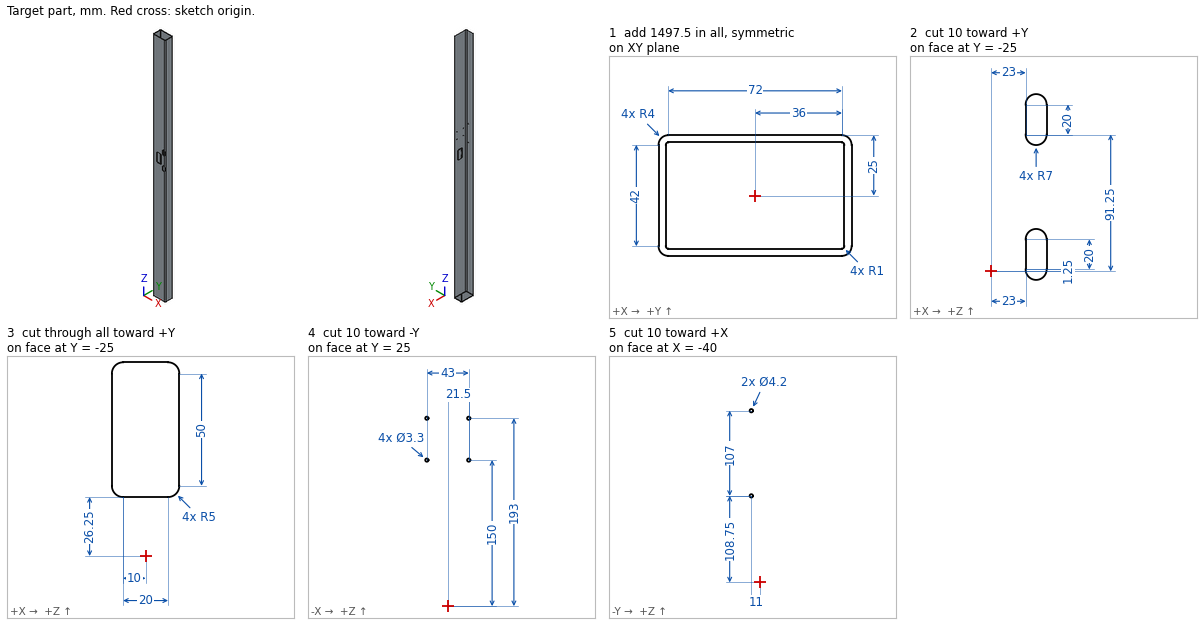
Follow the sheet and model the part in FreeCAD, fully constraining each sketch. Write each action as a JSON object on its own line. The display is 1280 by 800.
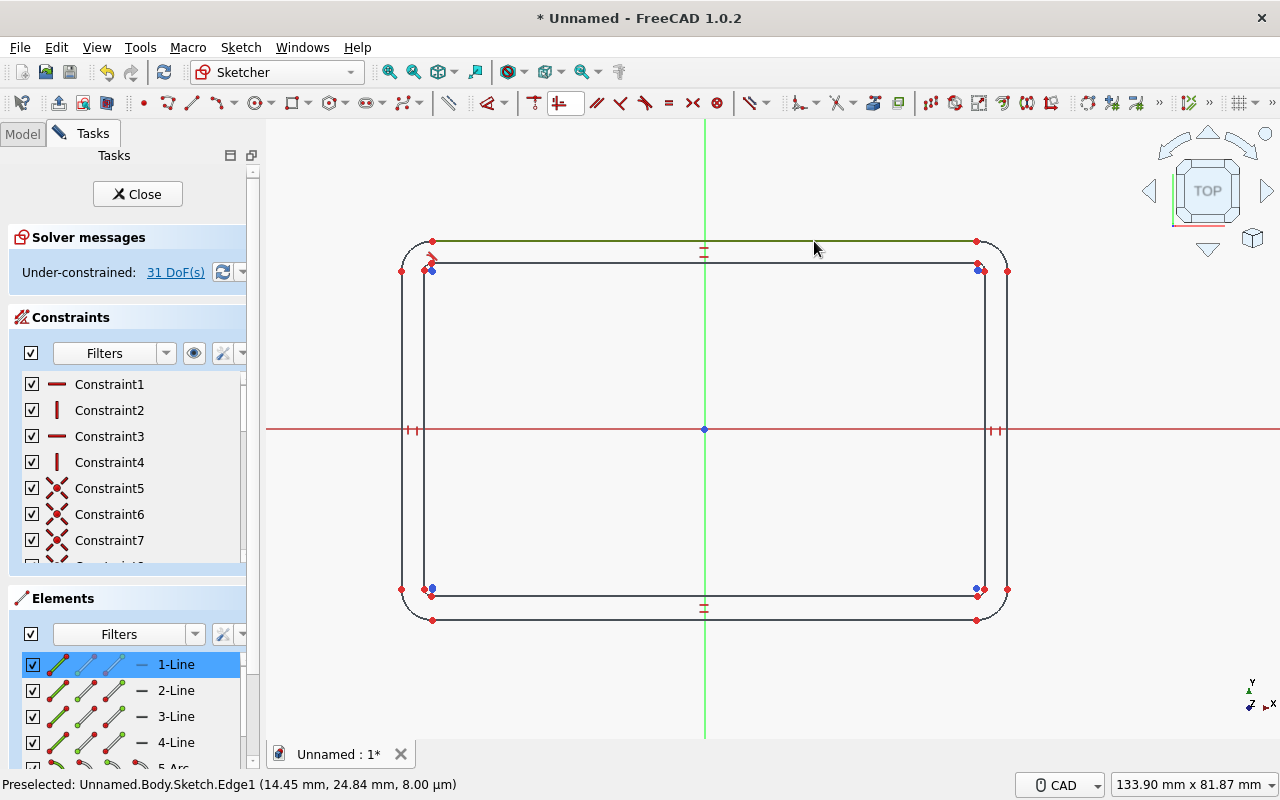
{"action": "left_click", "coordinate": [1005, 258]}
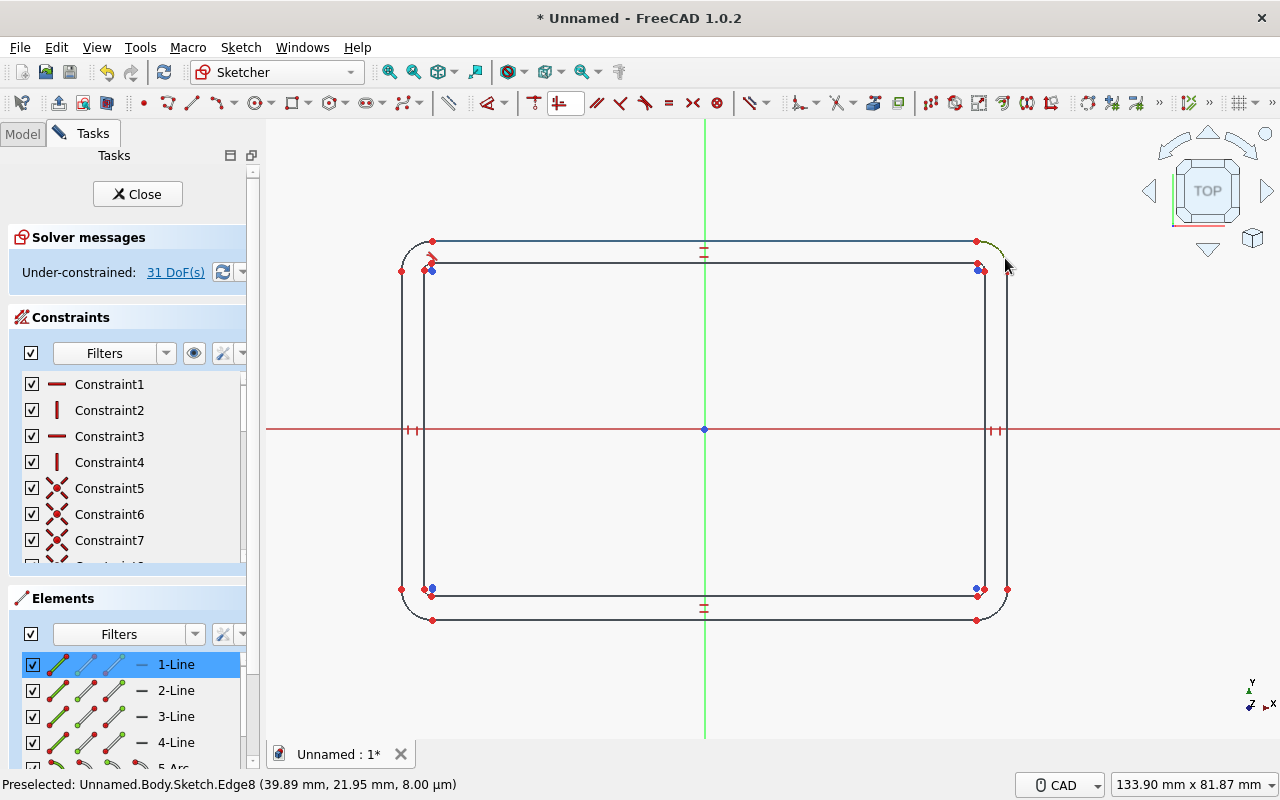
{"action": "left_click", "coordinate": [646, 104]}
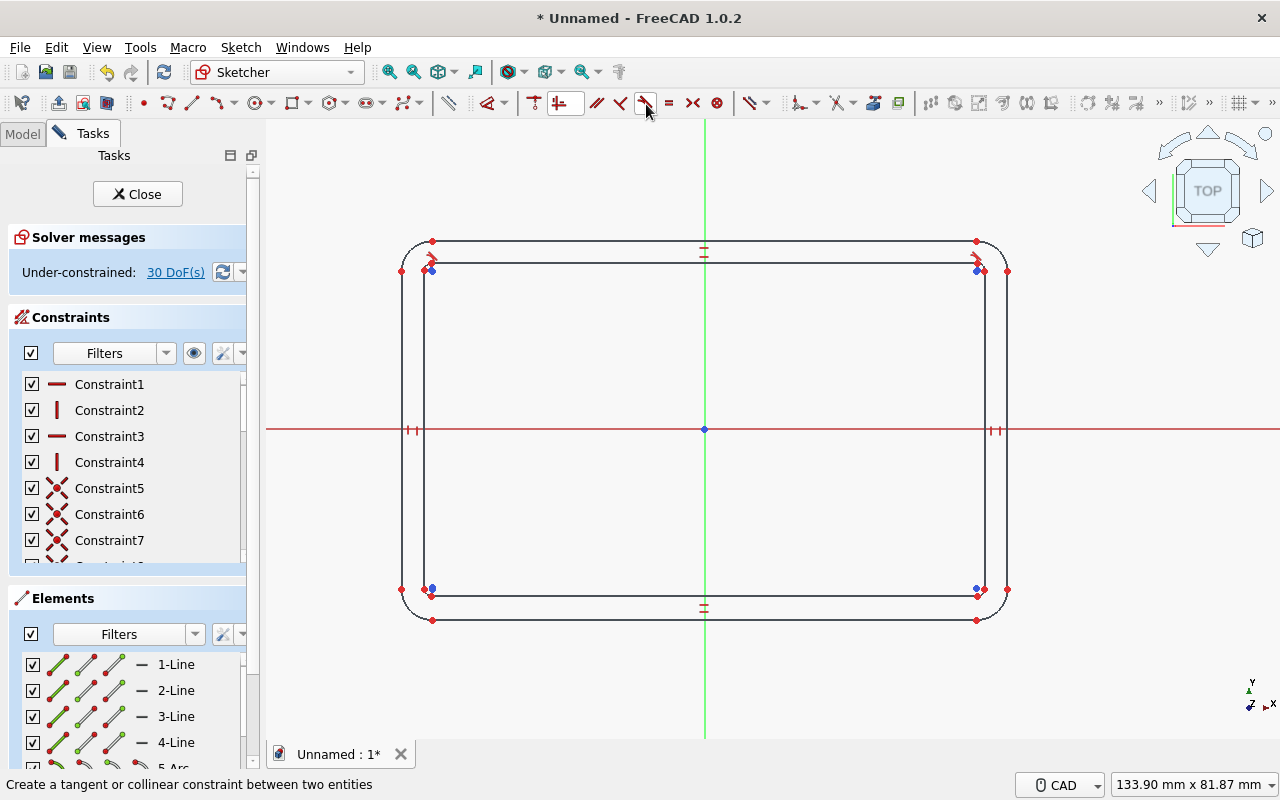
{"action": "left_click", "coordinate": [402, 367]}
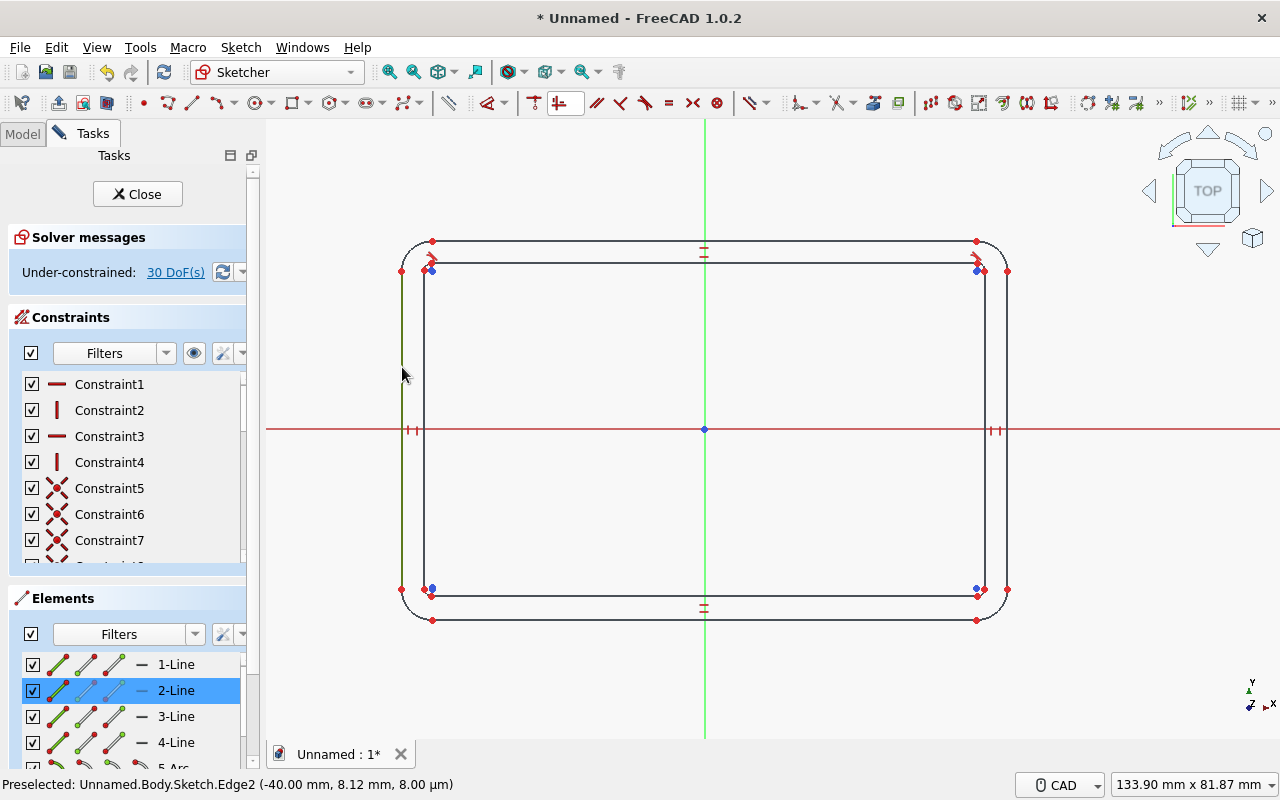
{"action": "left_click", "coordinate": [418, 245]}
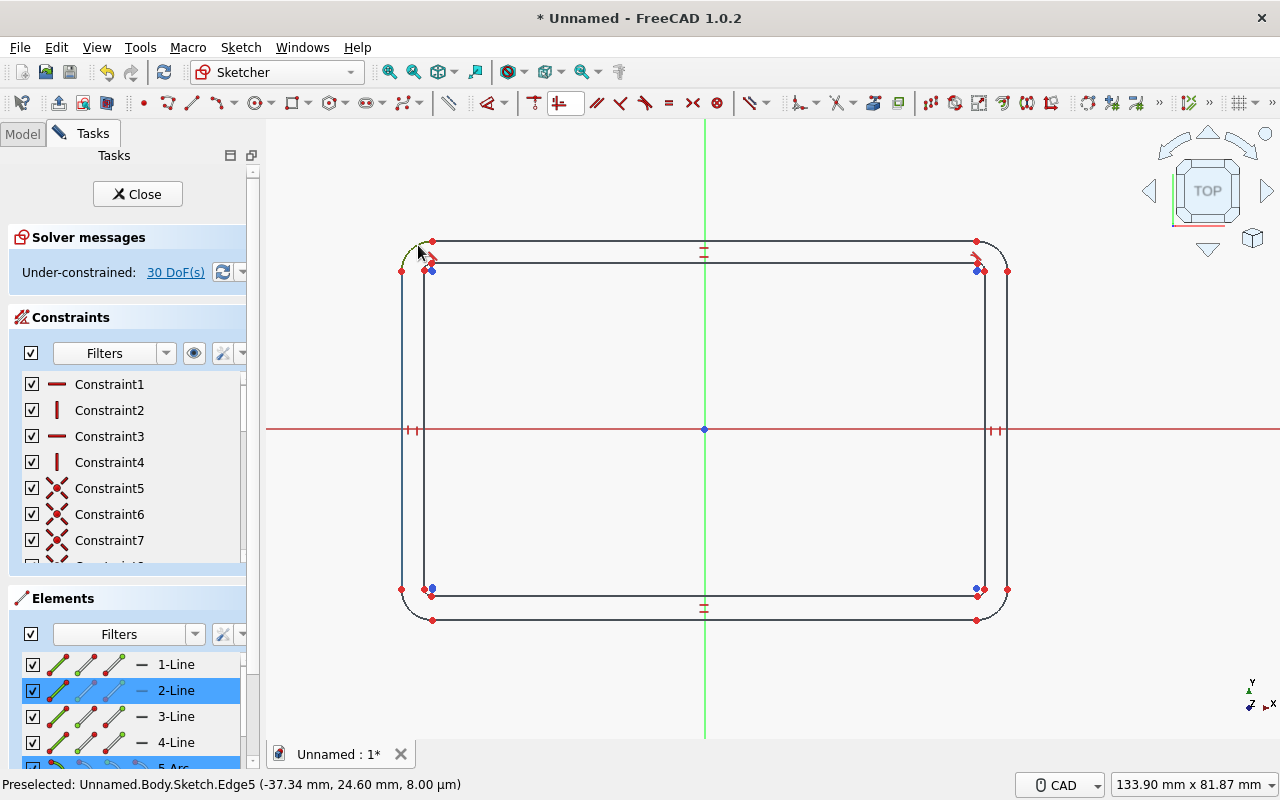
{"action": "key", "text": "t"}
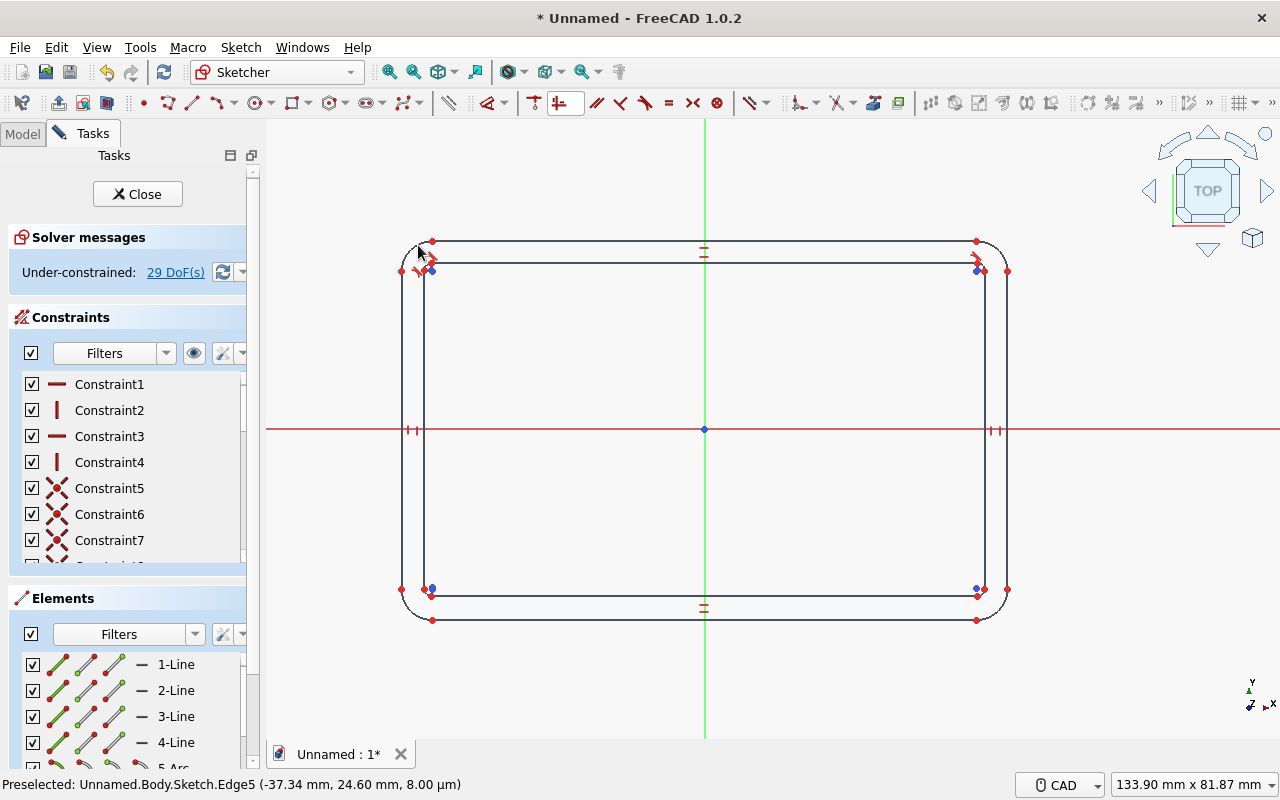
{"action": "left_click", "coordinate": [402, 367]}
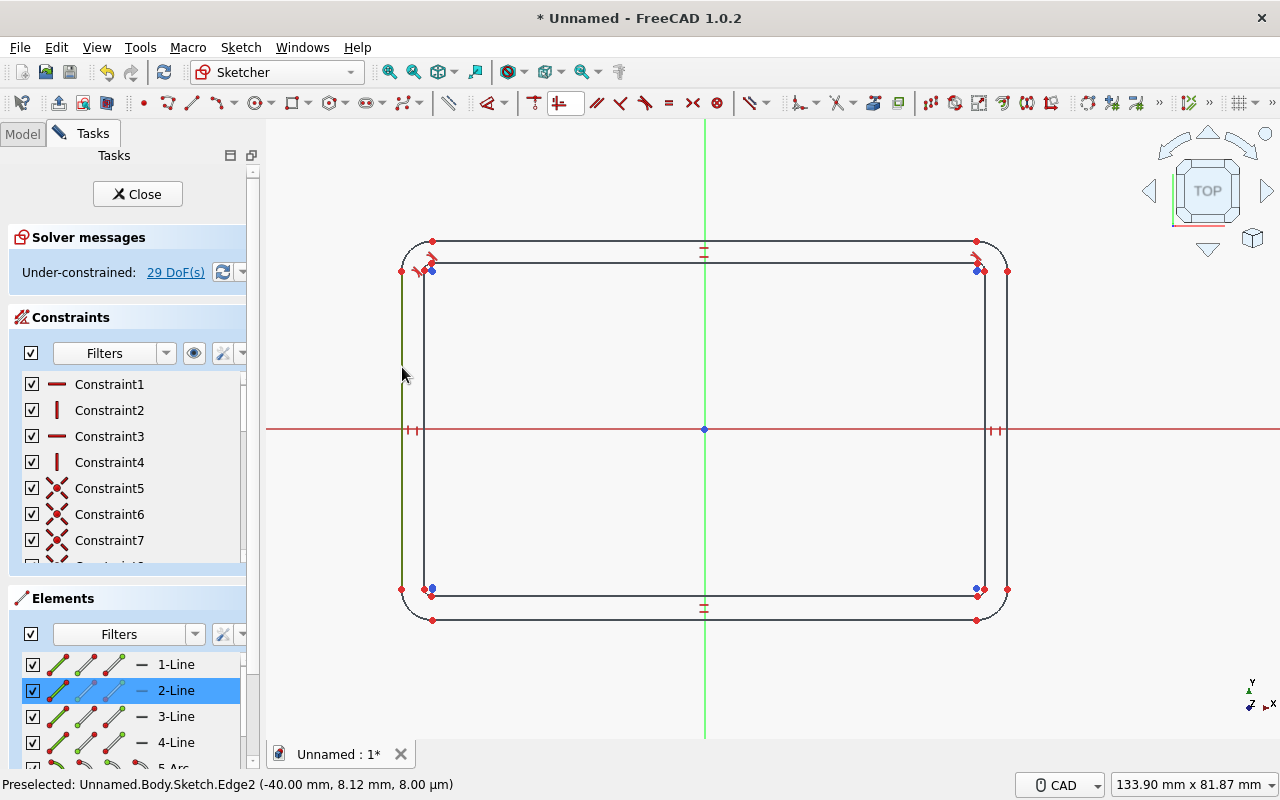
{"action": "left_click", "coordinate": [405, 603]}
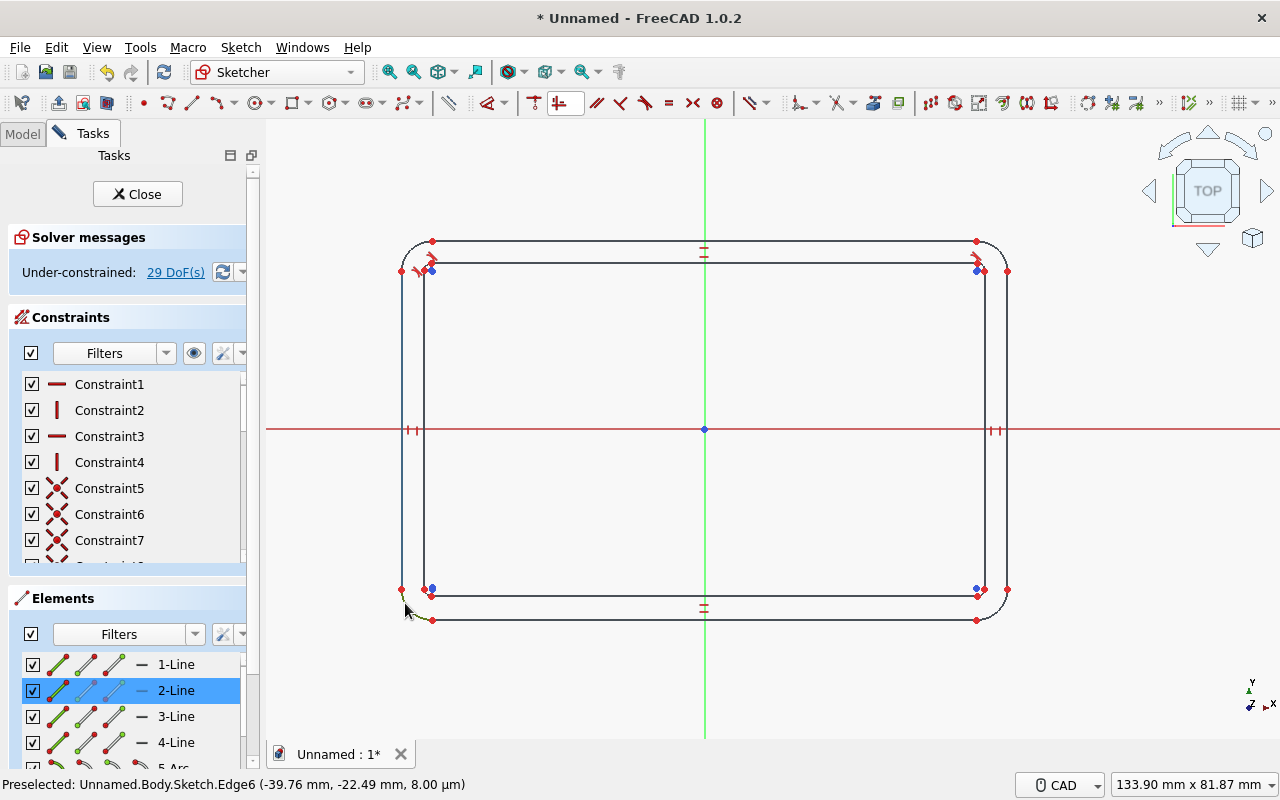
{"action": "key", "text": "t"}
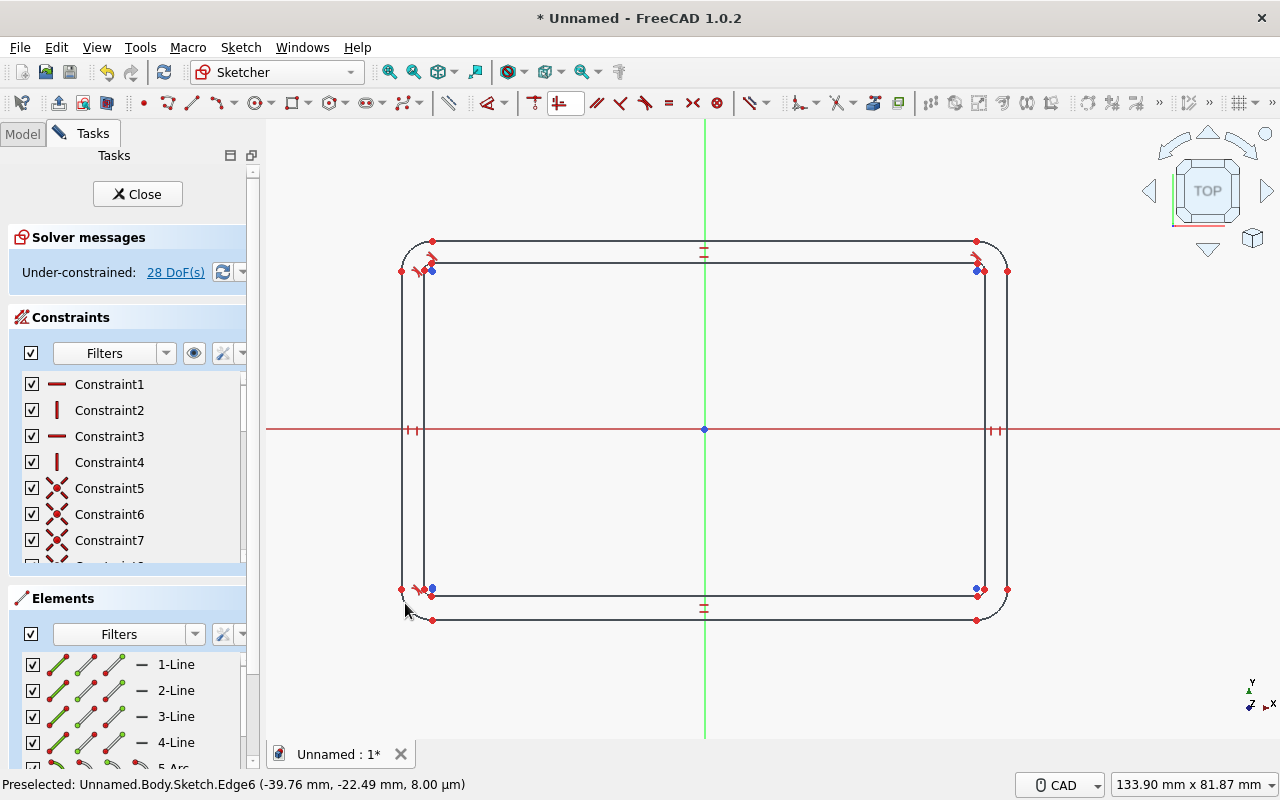
{"action": "left_click", "coordinate": [596, 620]}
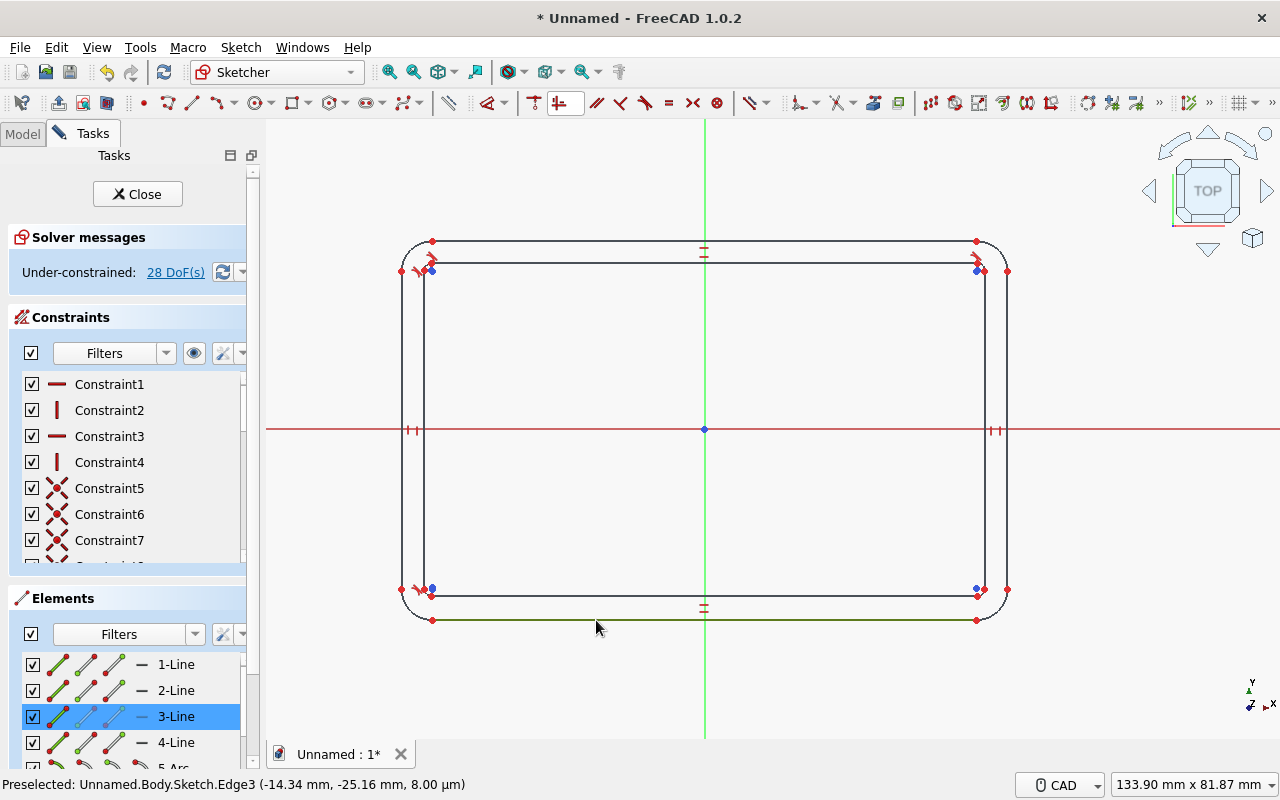
{"action": "left_click", "coordinate": [405, 603]}